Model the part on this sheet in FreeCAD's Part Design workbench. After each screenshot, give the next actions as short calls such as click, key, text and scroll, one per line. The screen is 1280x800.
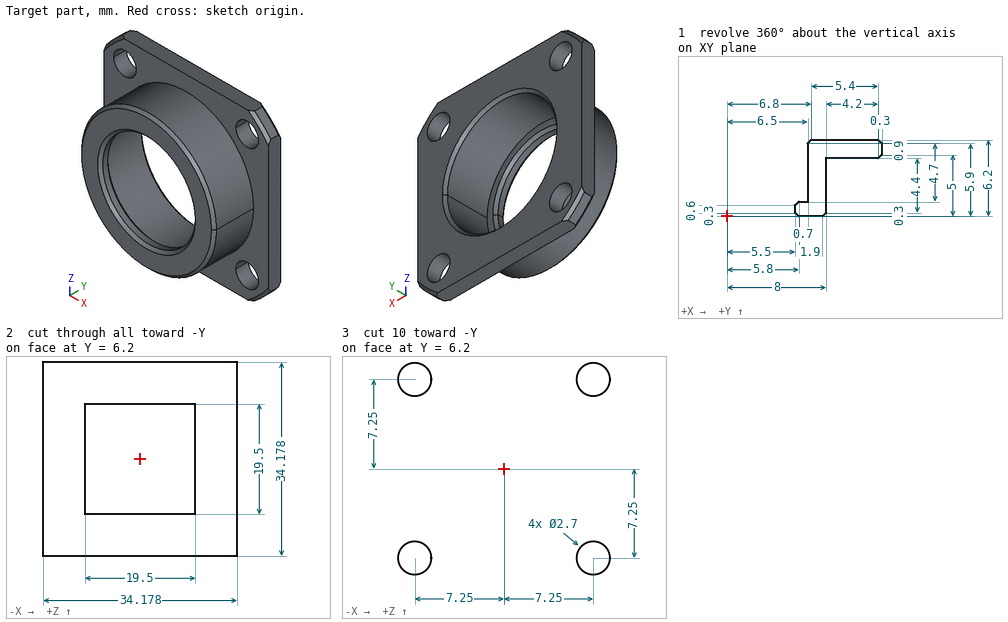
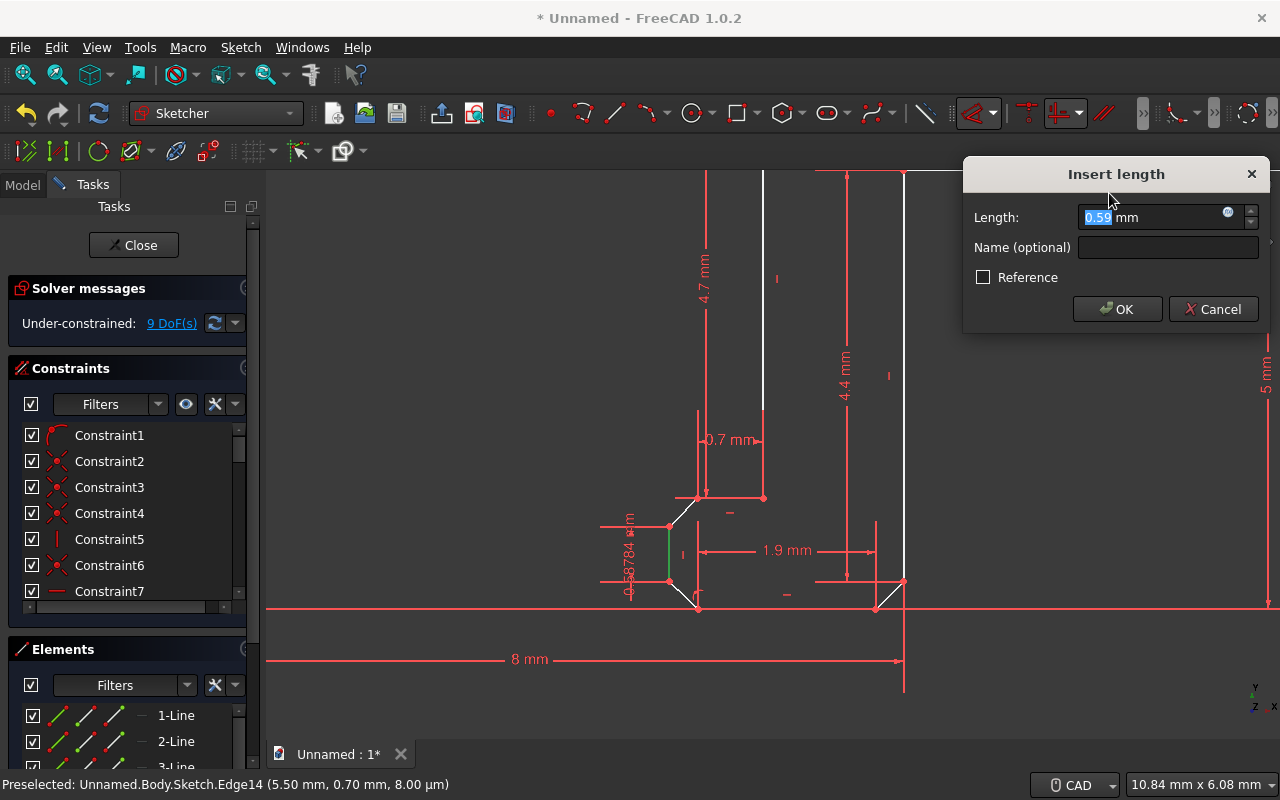
text(0.6)
key(Return)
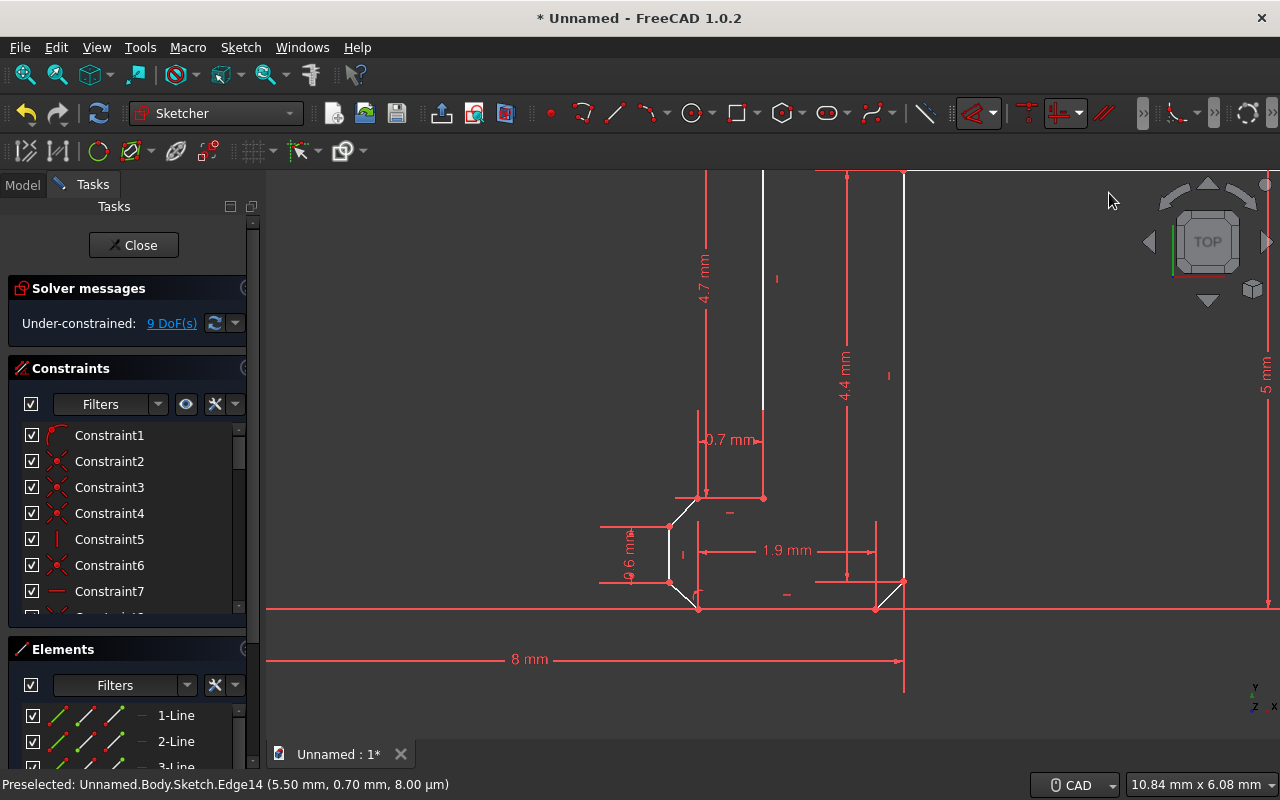
click(669, 583)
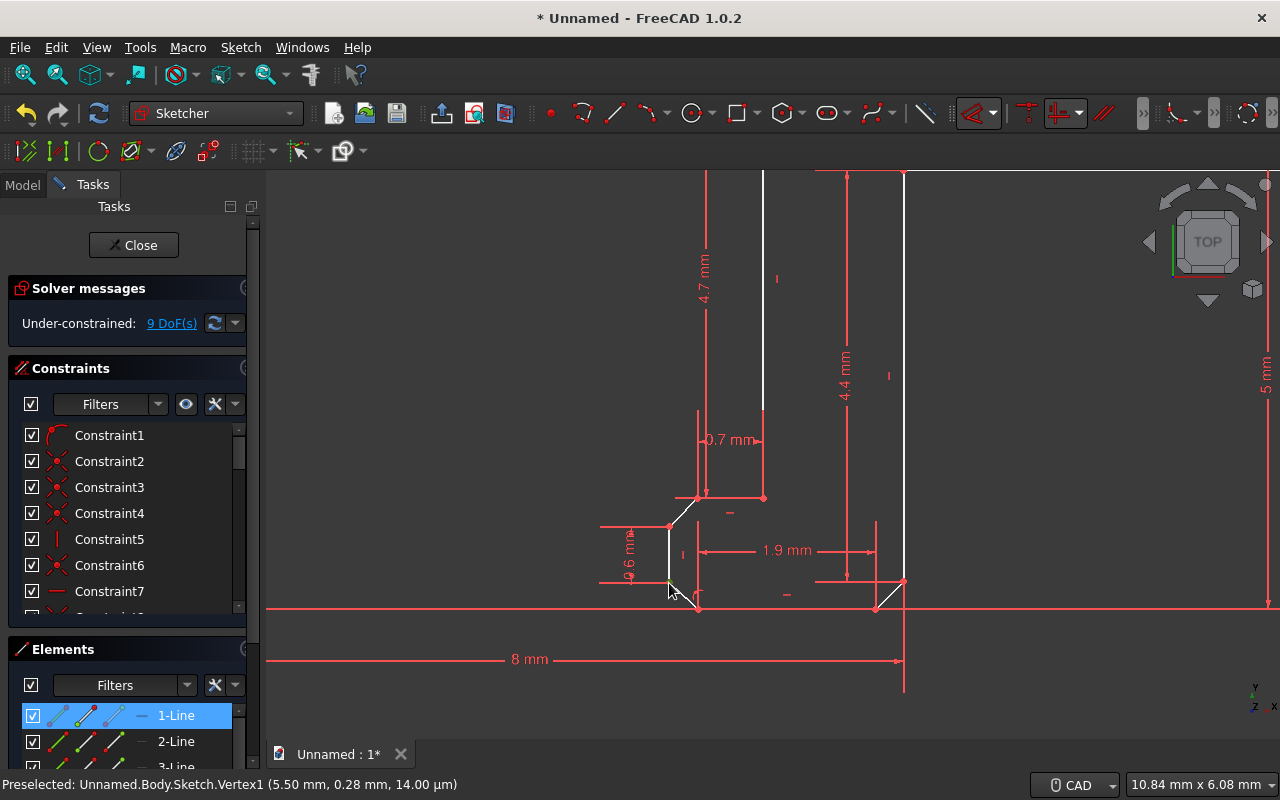
click(996, 114)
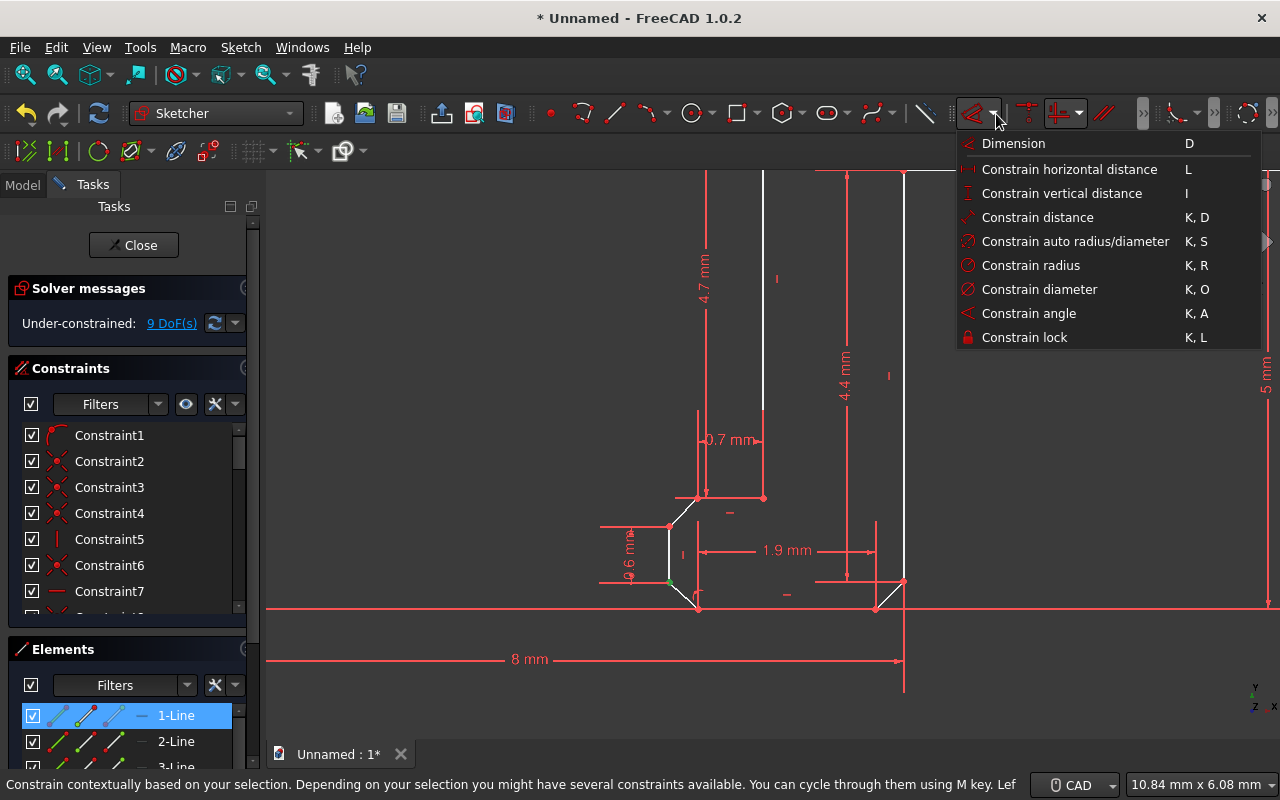
click(1109, 169)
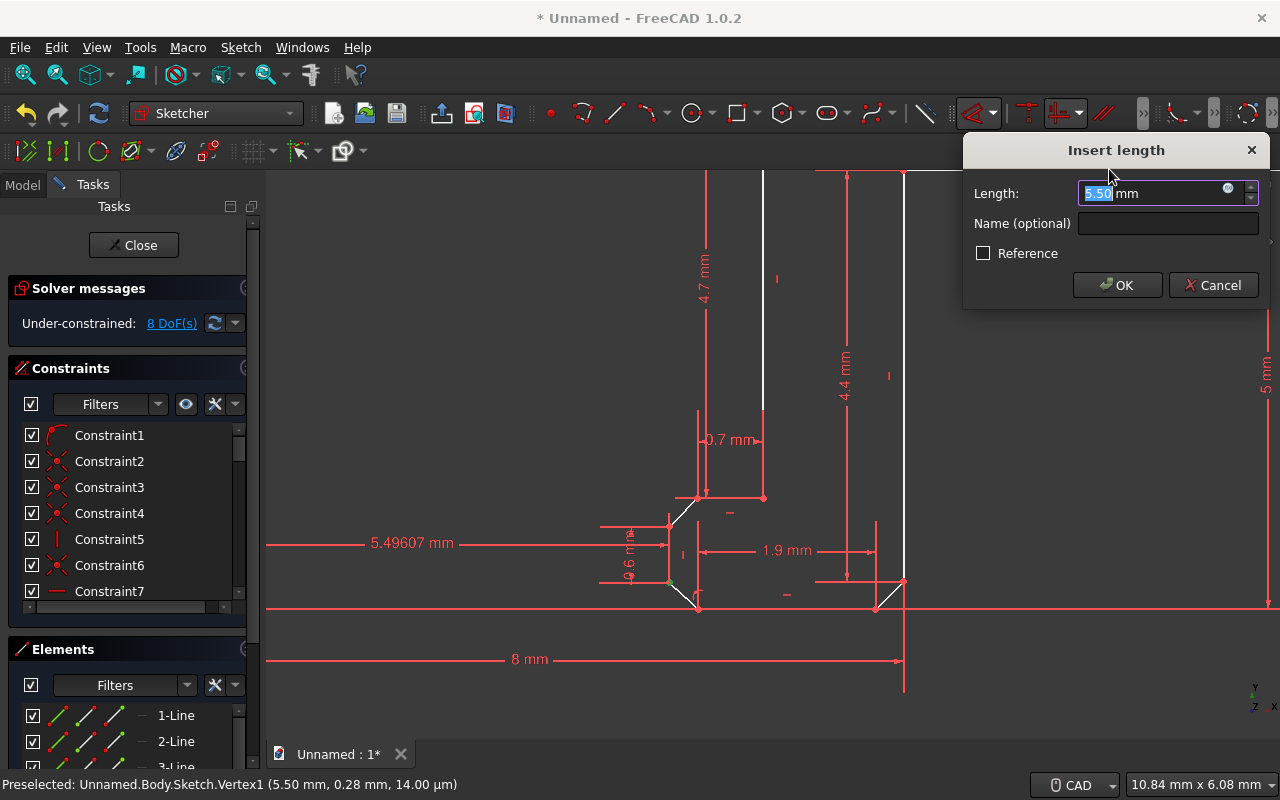
text(5.5)
key(Return)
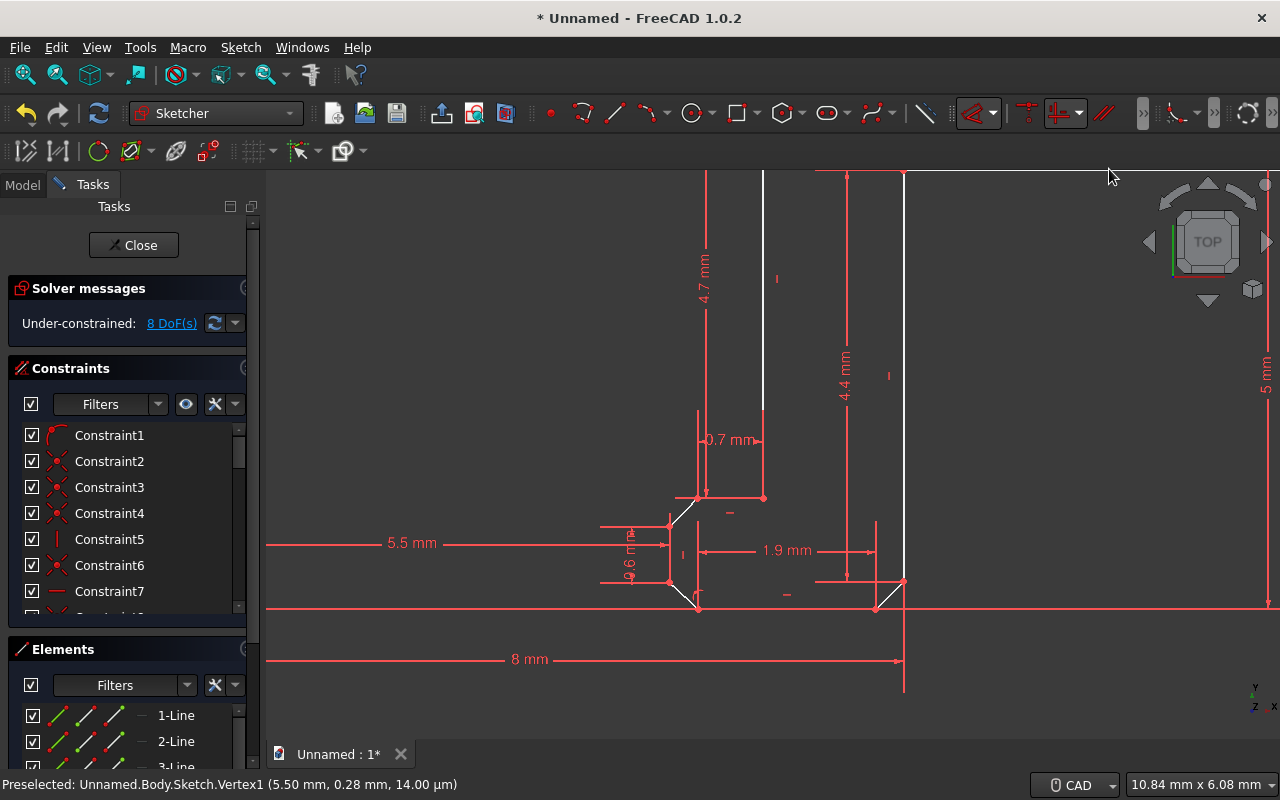
scroll(670, 583, up, 2)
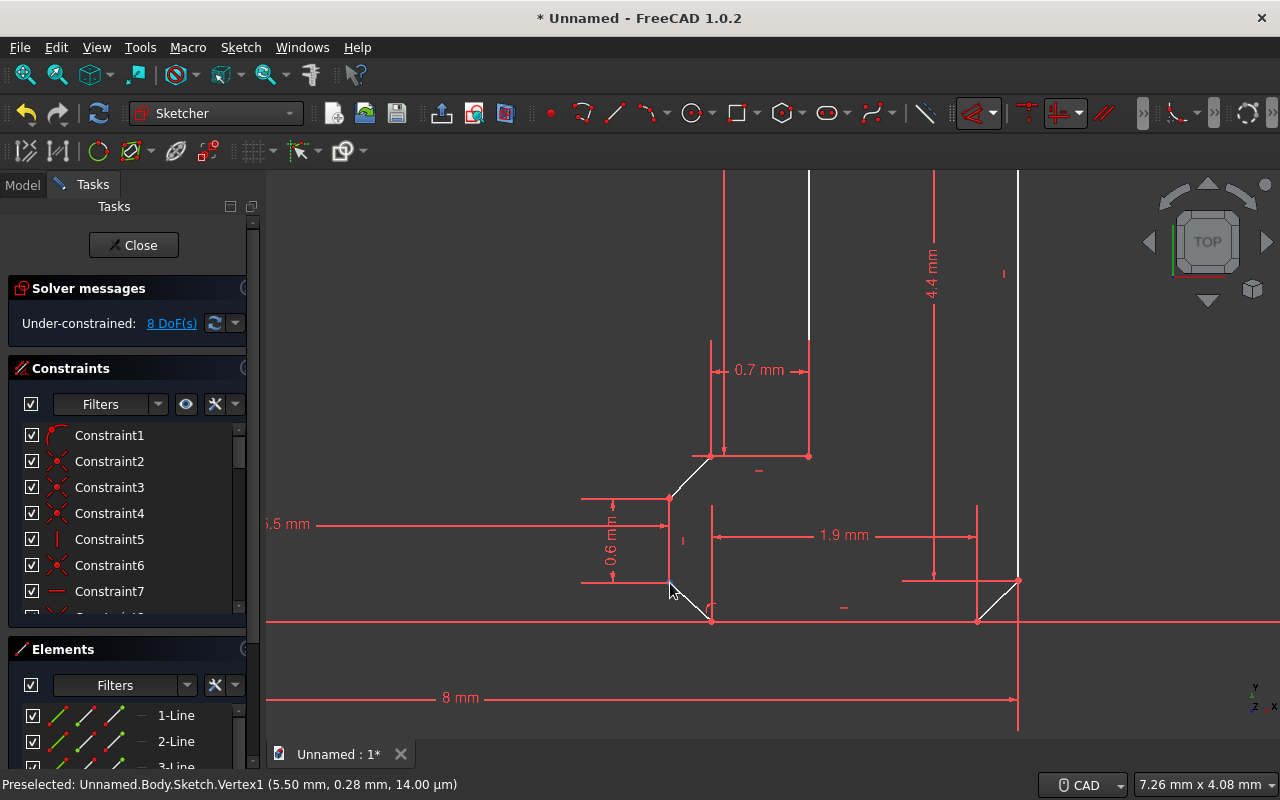
click(669, 583)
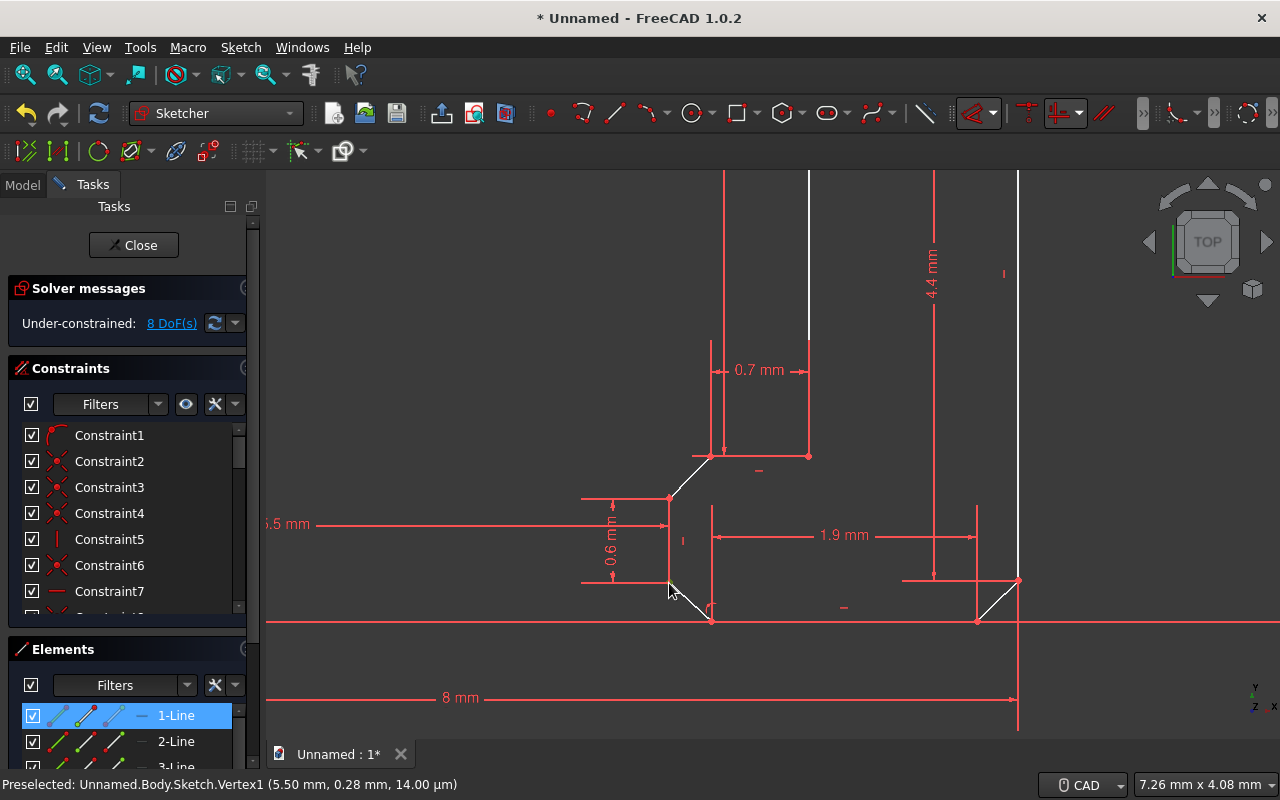
click(996, 114)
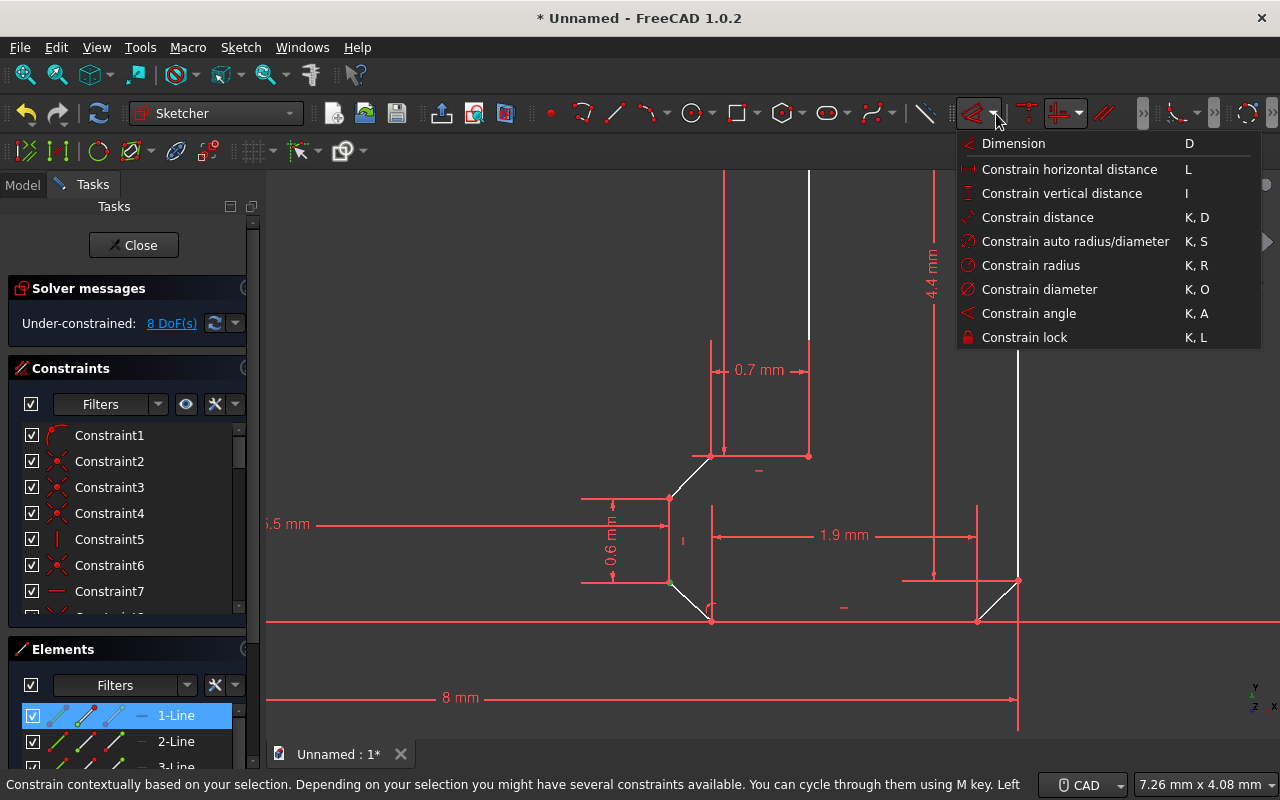
click(1109, 193)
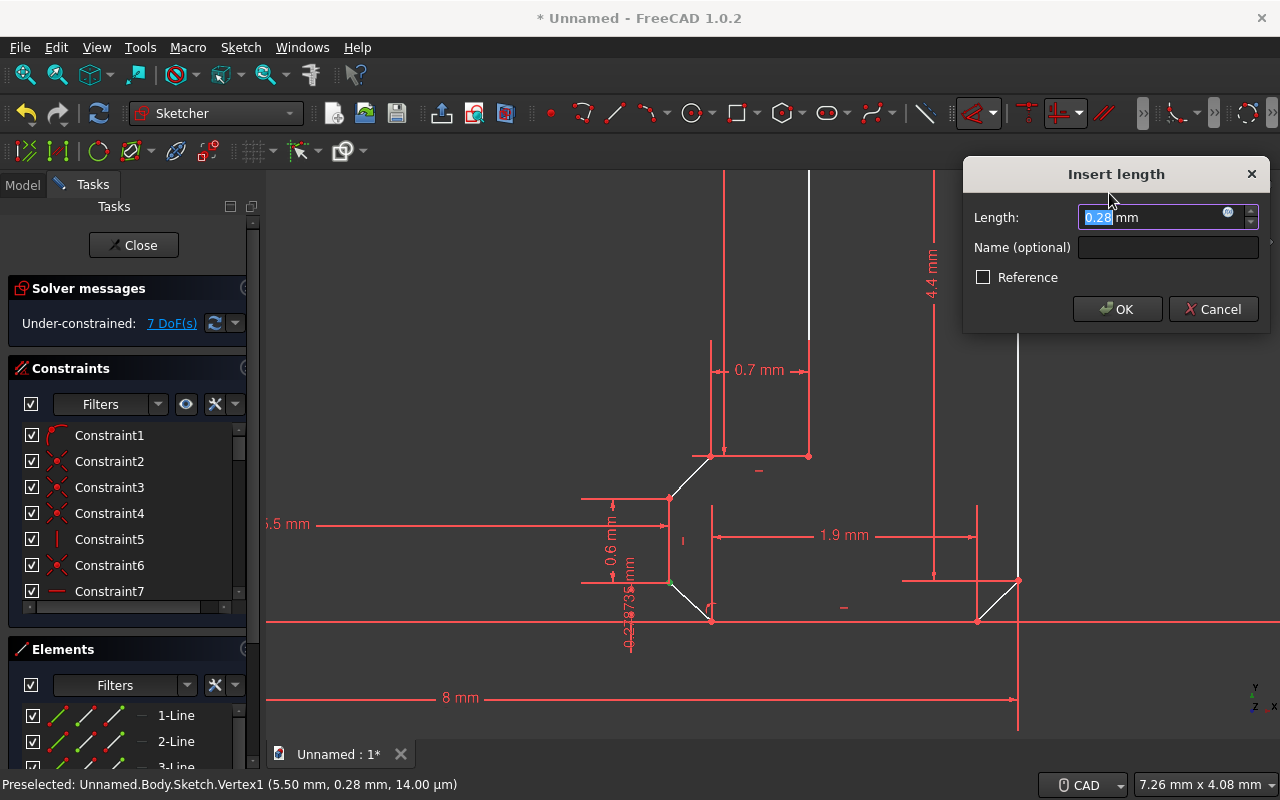
text(0.3)
key(Return)